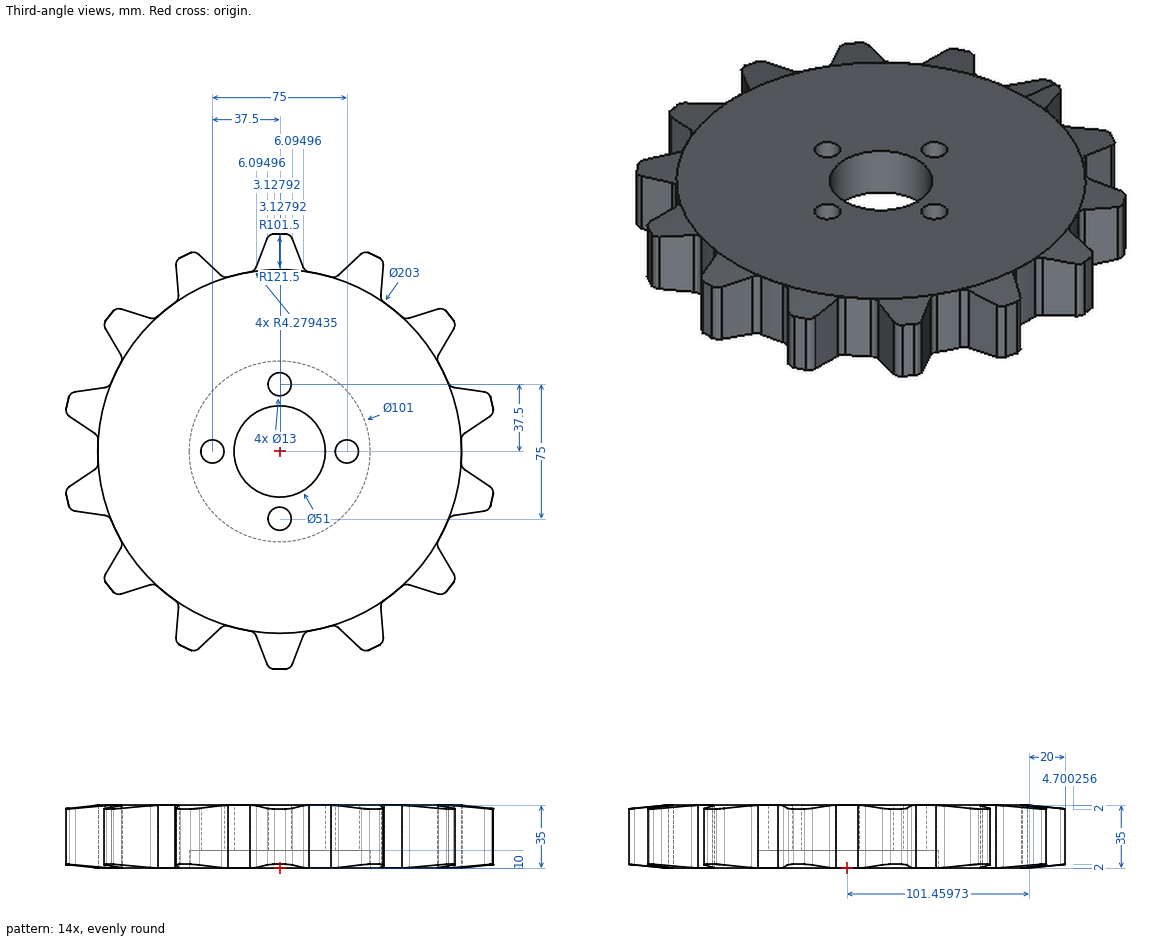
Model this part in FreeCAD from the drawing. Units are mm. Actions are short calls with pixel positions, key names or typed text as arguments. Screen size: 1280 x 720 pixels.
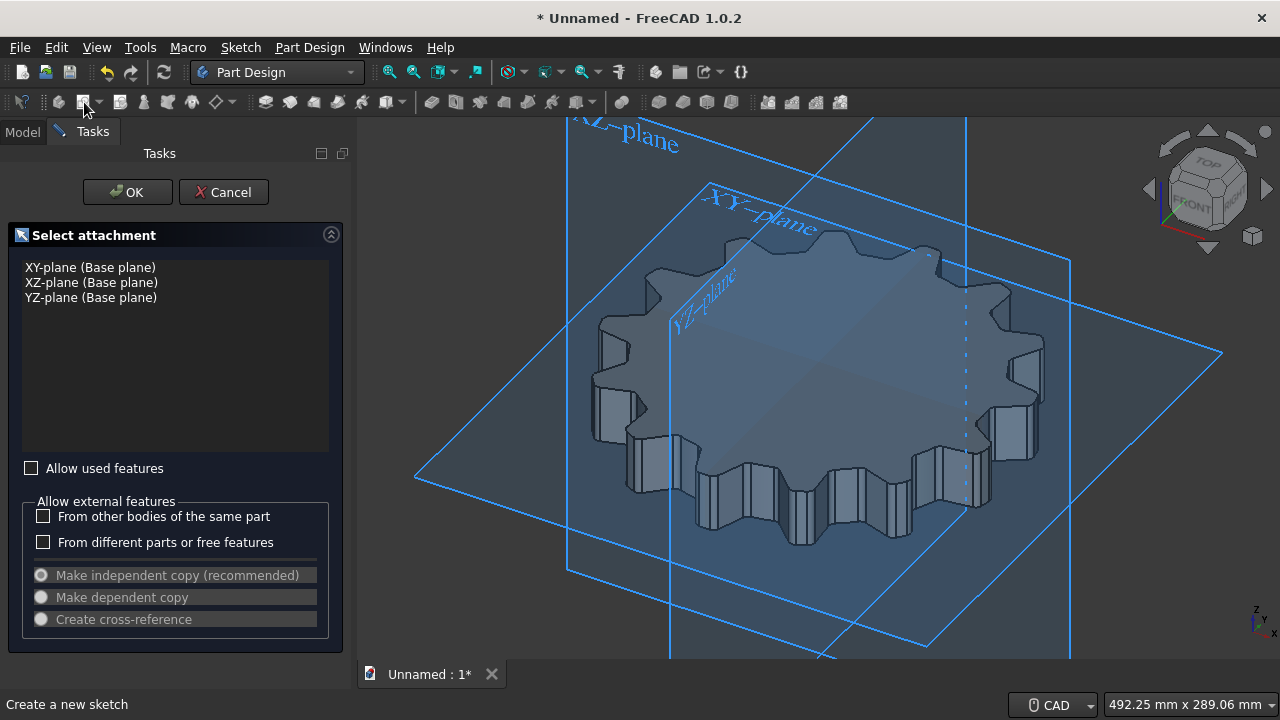
click(82, 298)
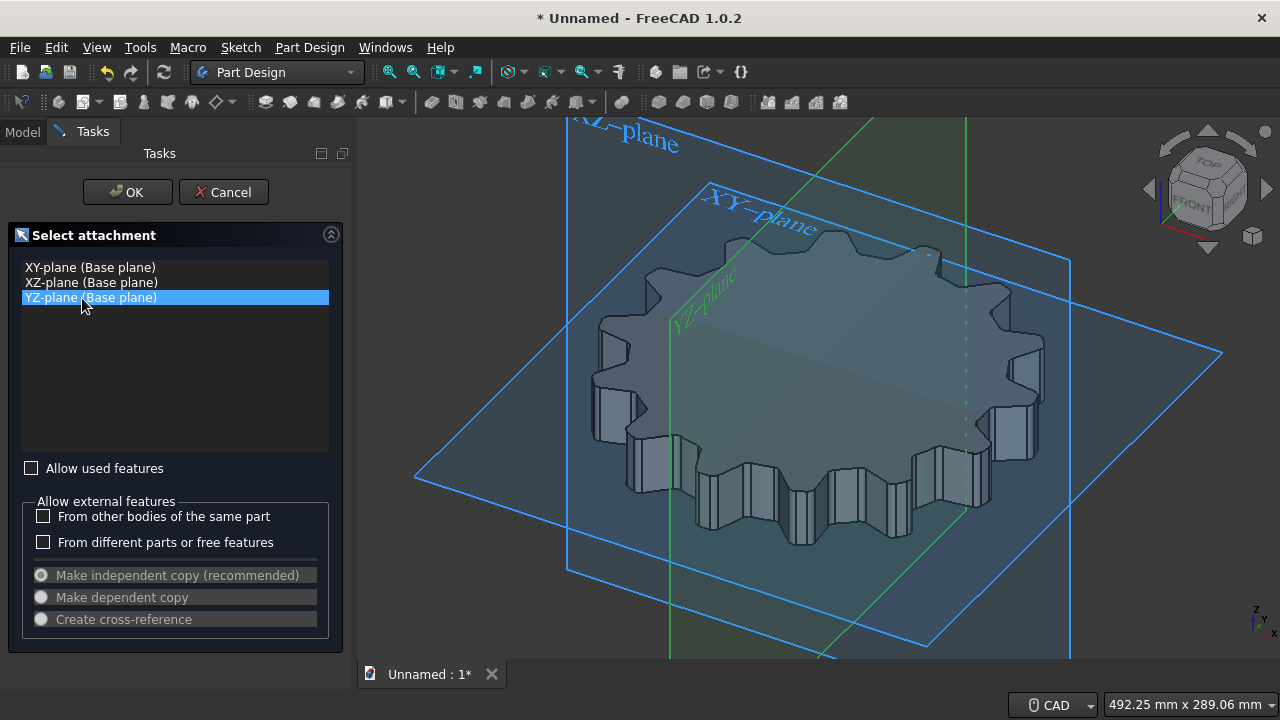
click(128, 192)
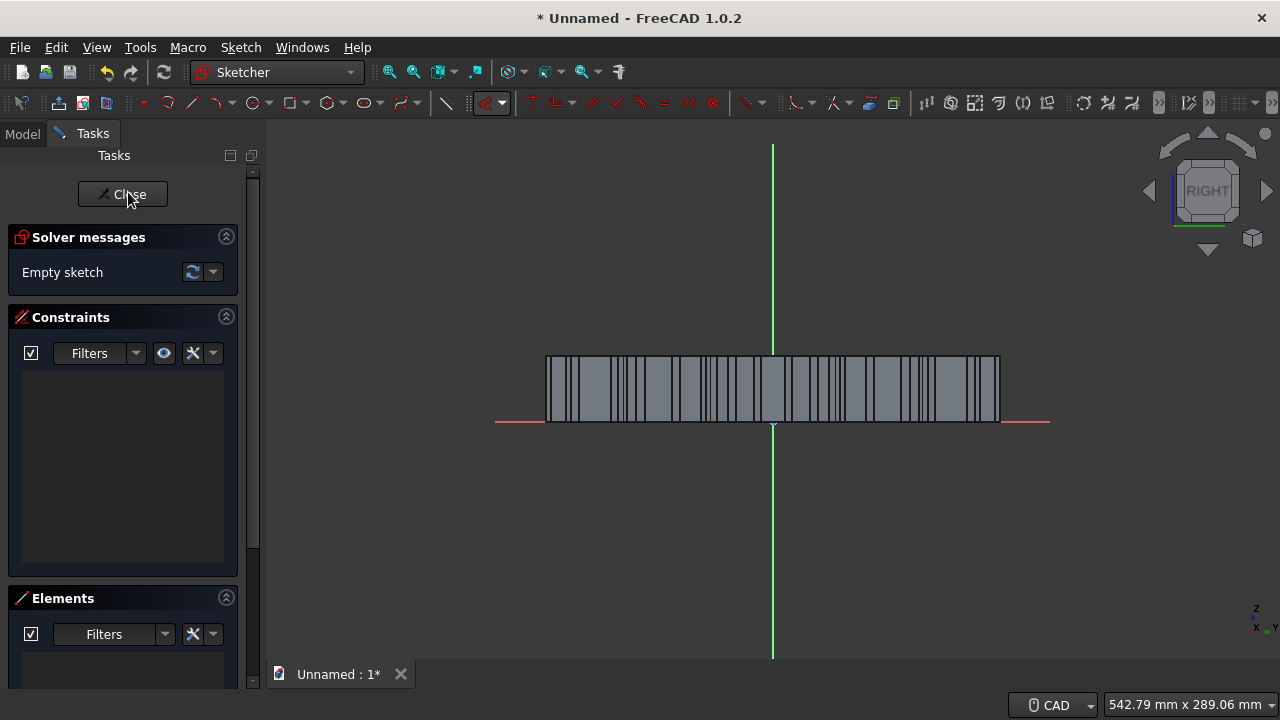
click(108, 104)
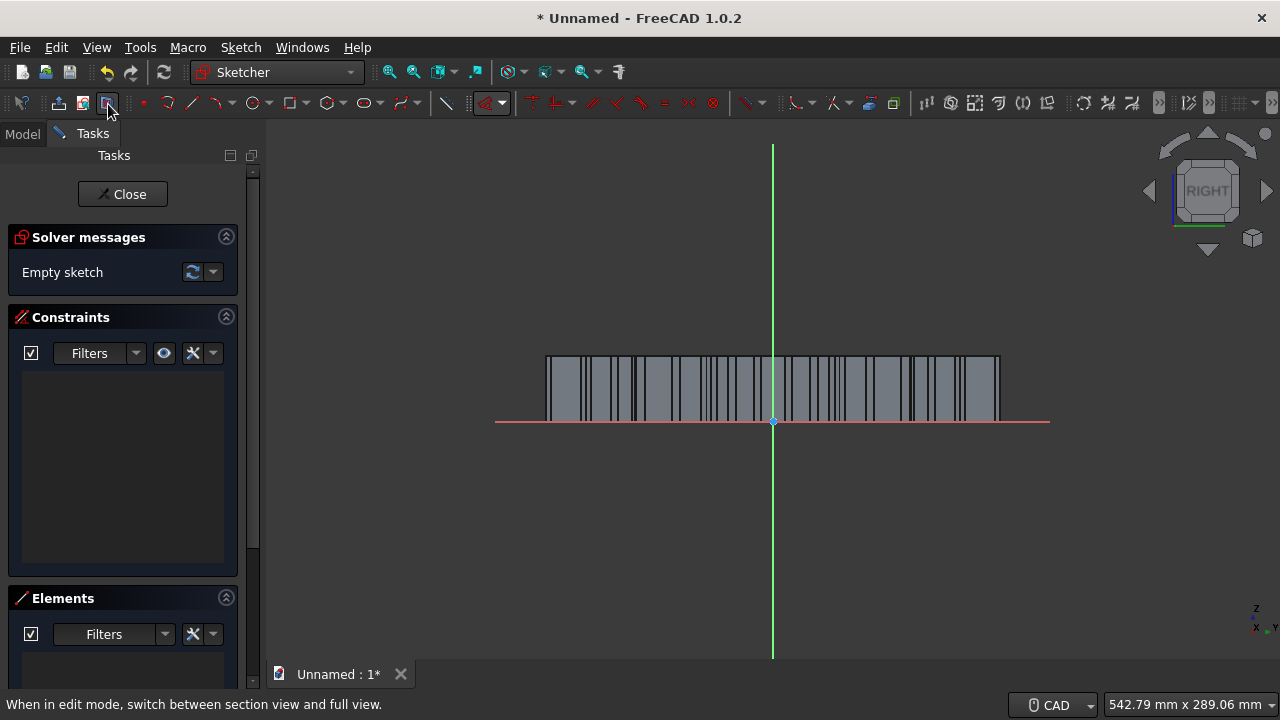
scroll(1057, 389, up, 8)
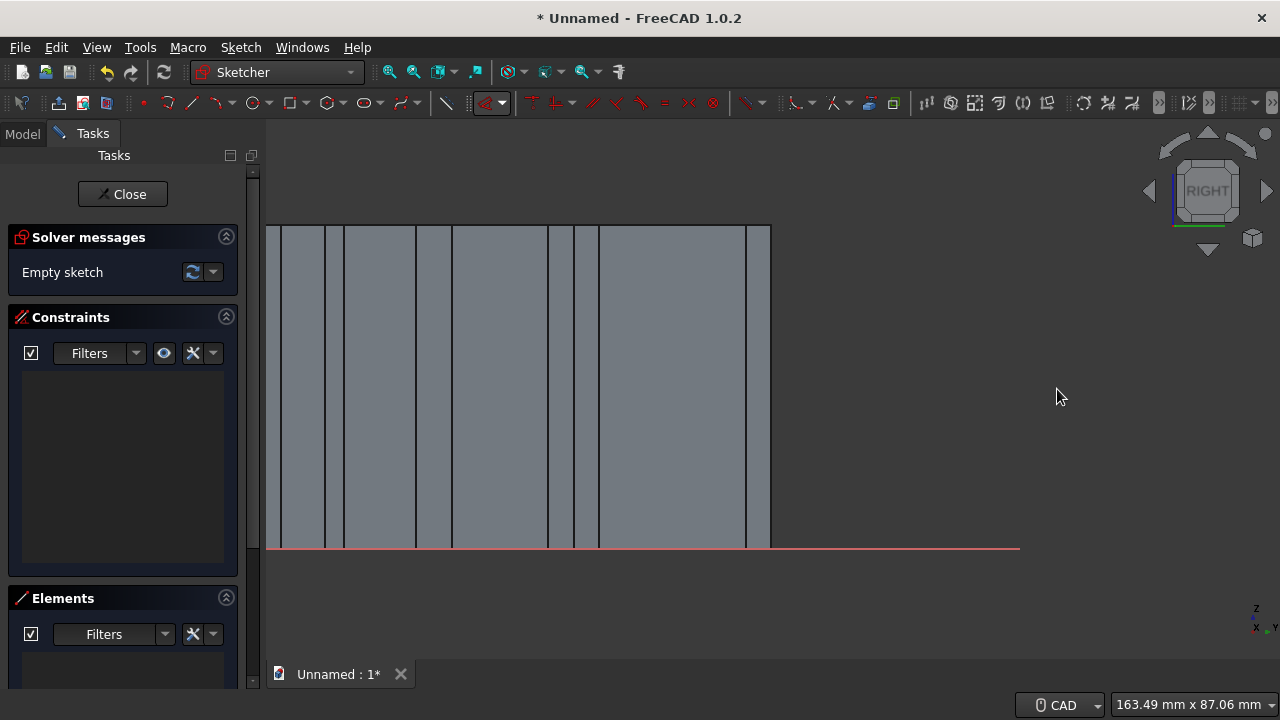
click(168, 104)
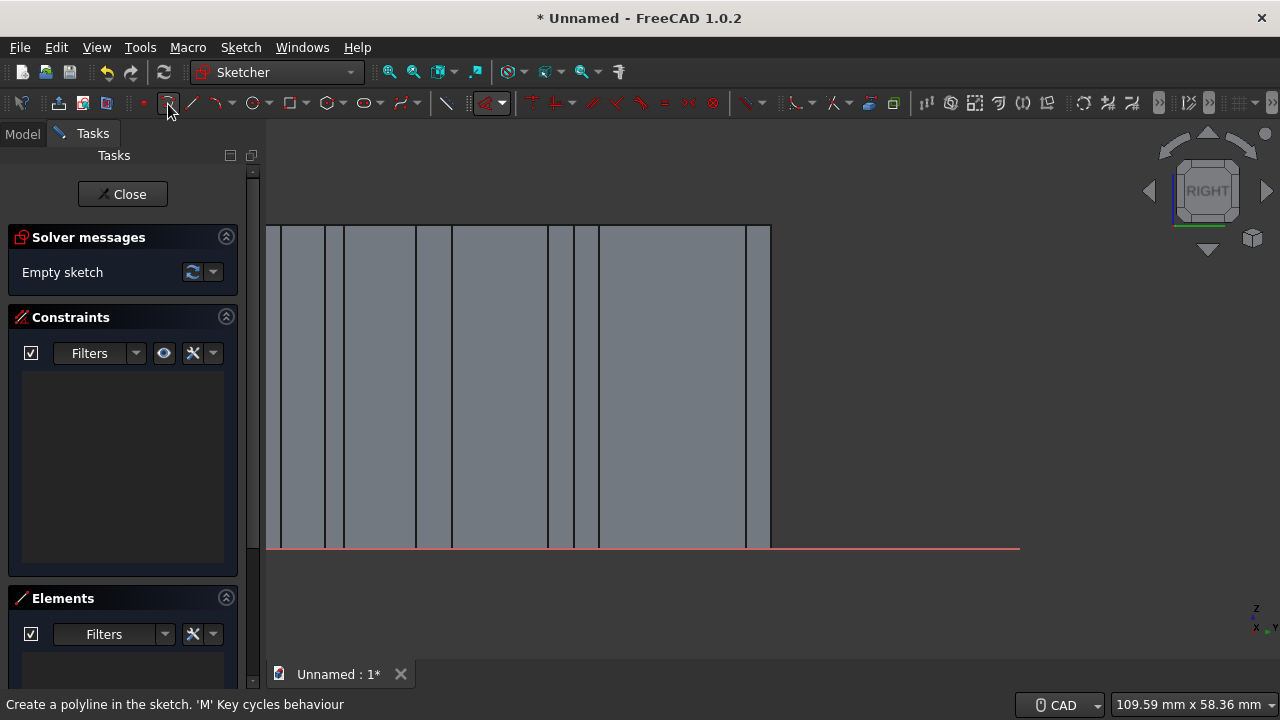
click(586, 225)
click(771, 244)
click(815, 244)
click(815, 225)
click(586, 226)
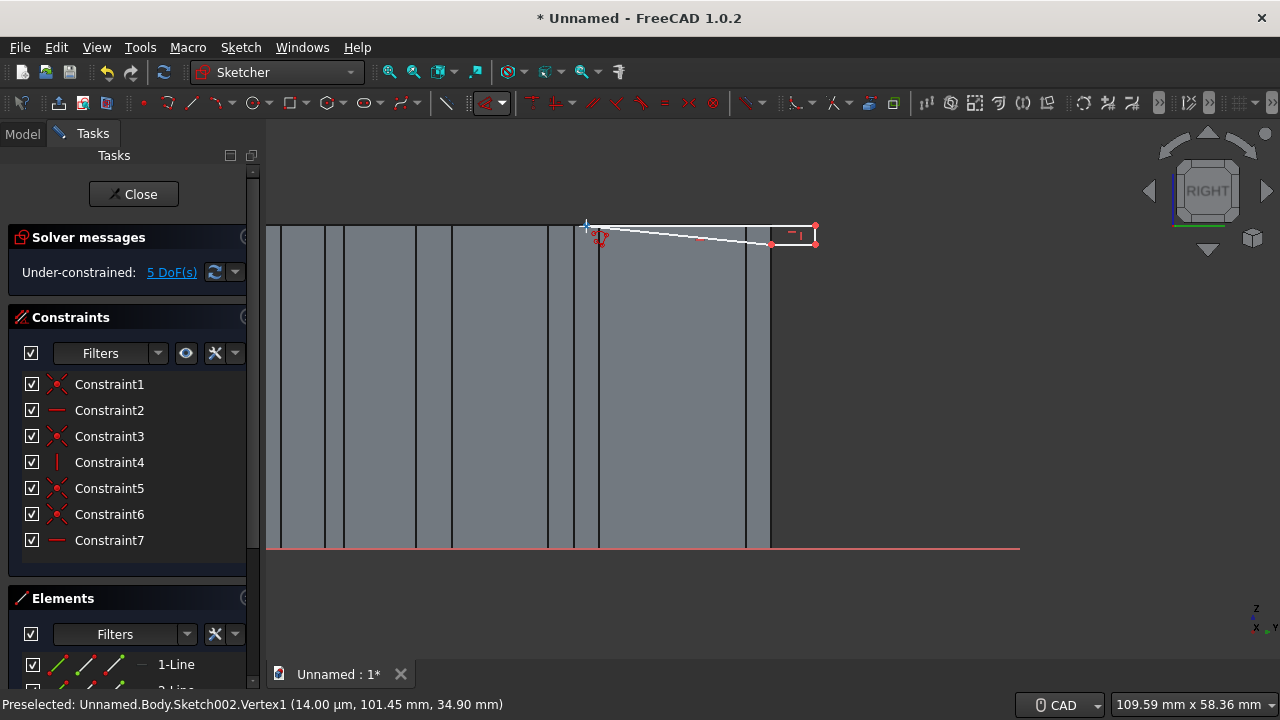
click(586, 549)
click(815, 540)
click(815, 530)
click(771, 530)
click(586, 549)
key(Escape)
key(Escape)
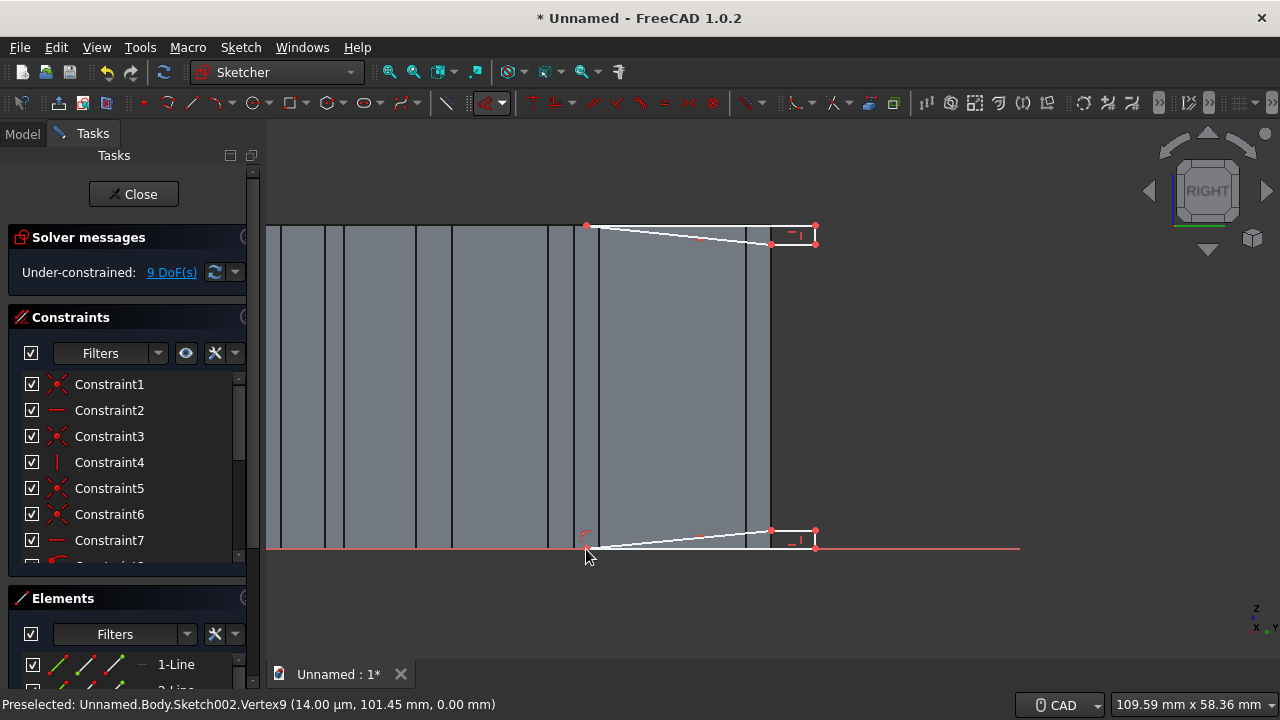
scroll(815, 235, up, 4)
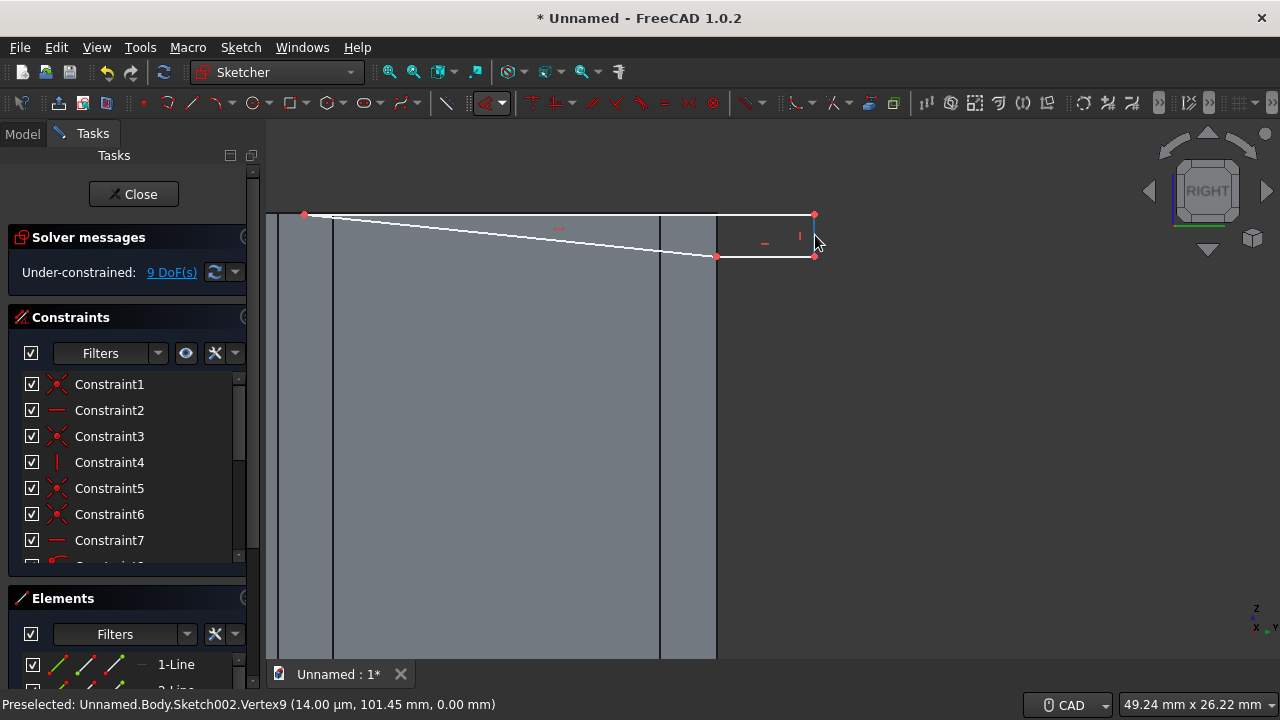
click(814, 236)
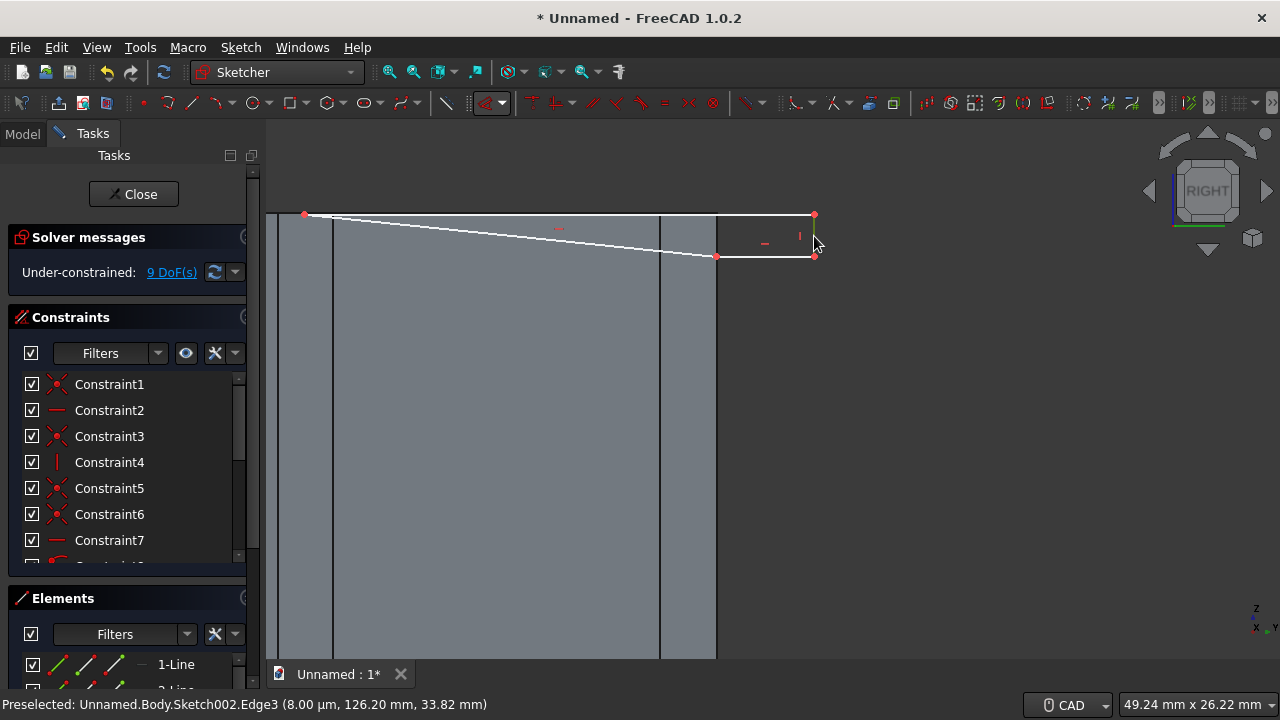
key(i)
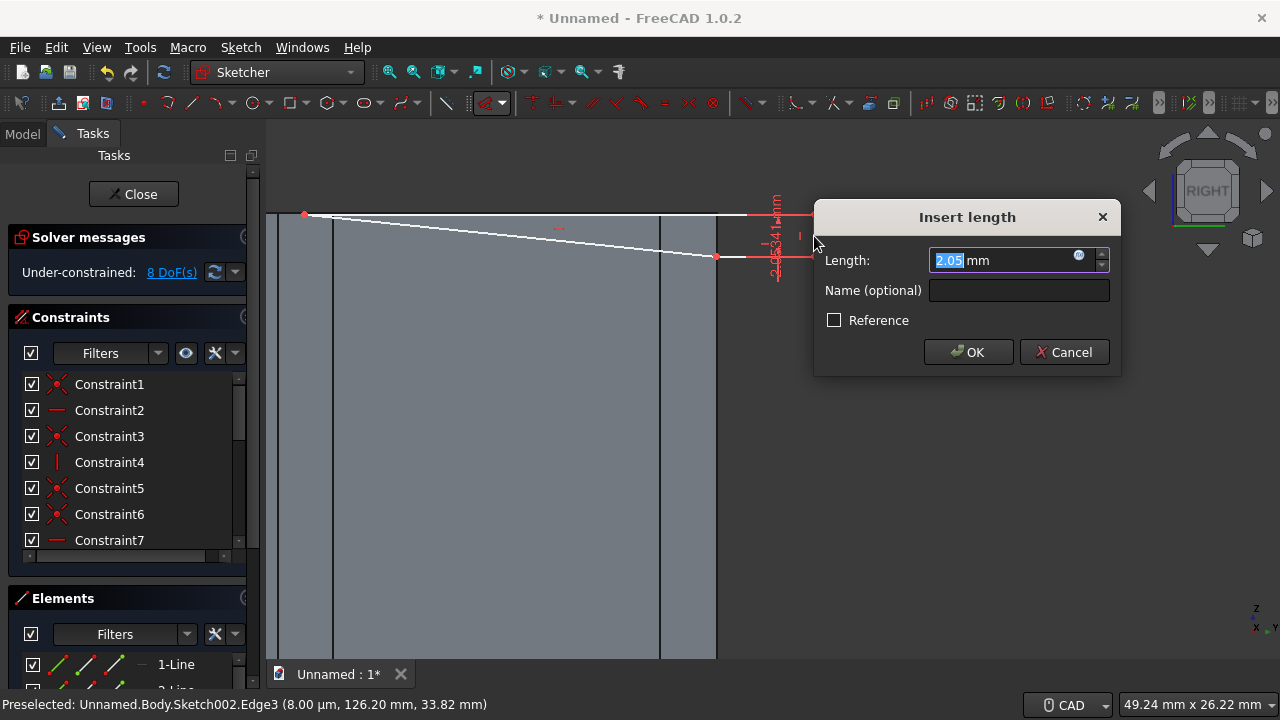
text(2)
key(Return)